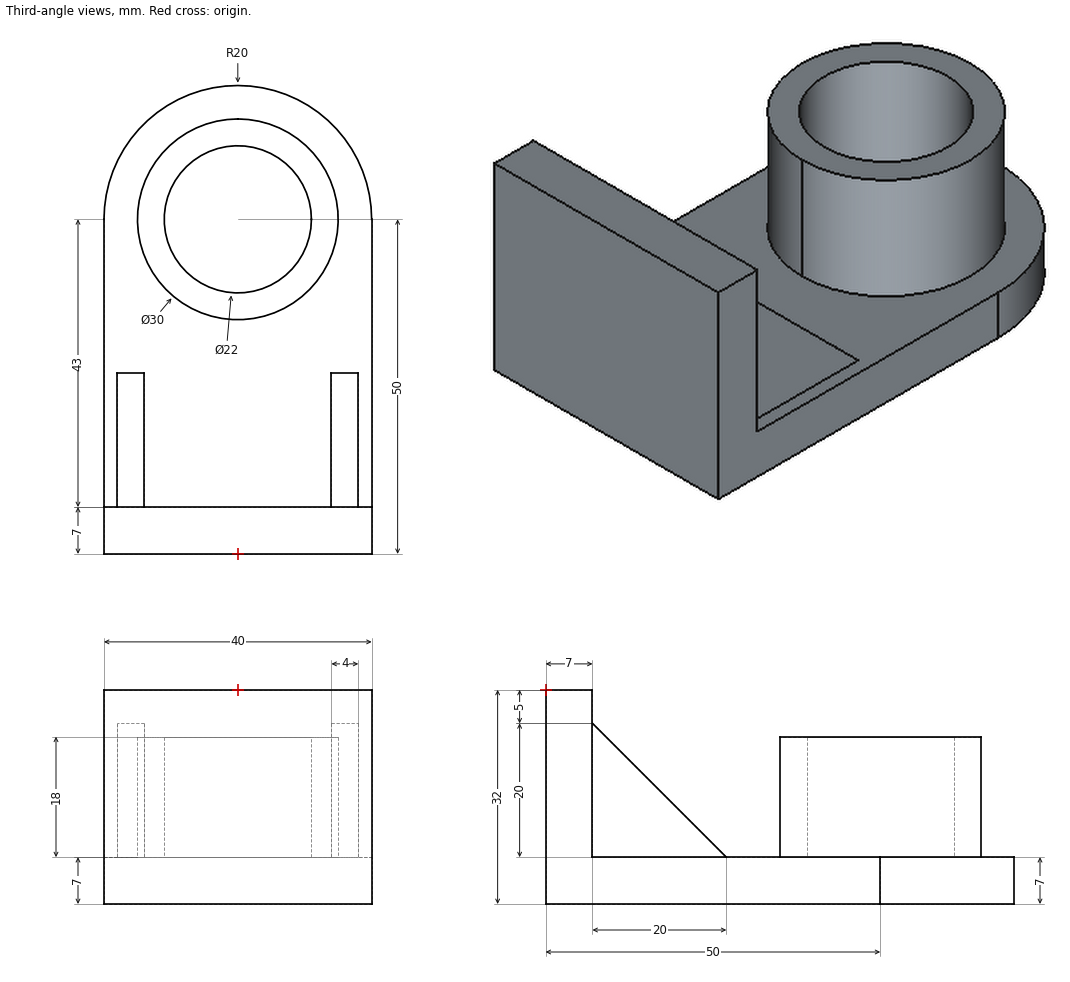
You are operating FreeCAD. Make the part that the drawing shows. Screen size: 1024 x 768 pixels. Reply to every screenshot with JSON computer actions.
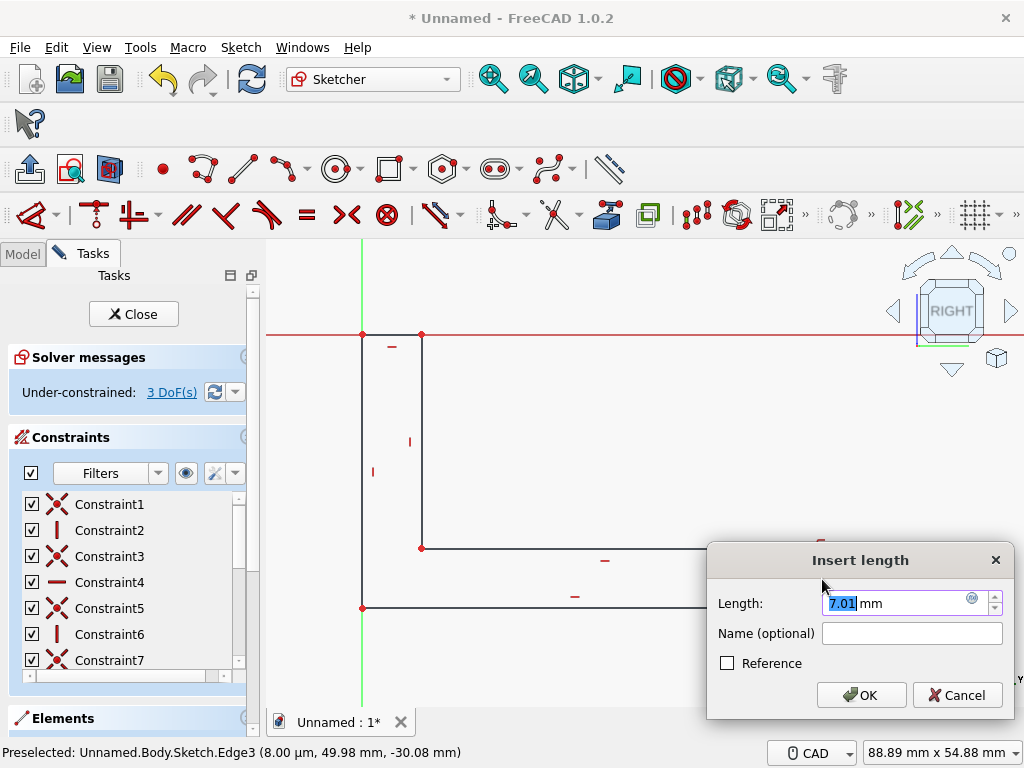
{"action": "type", "text": "7"}
{"action": "key", "text": "Return"}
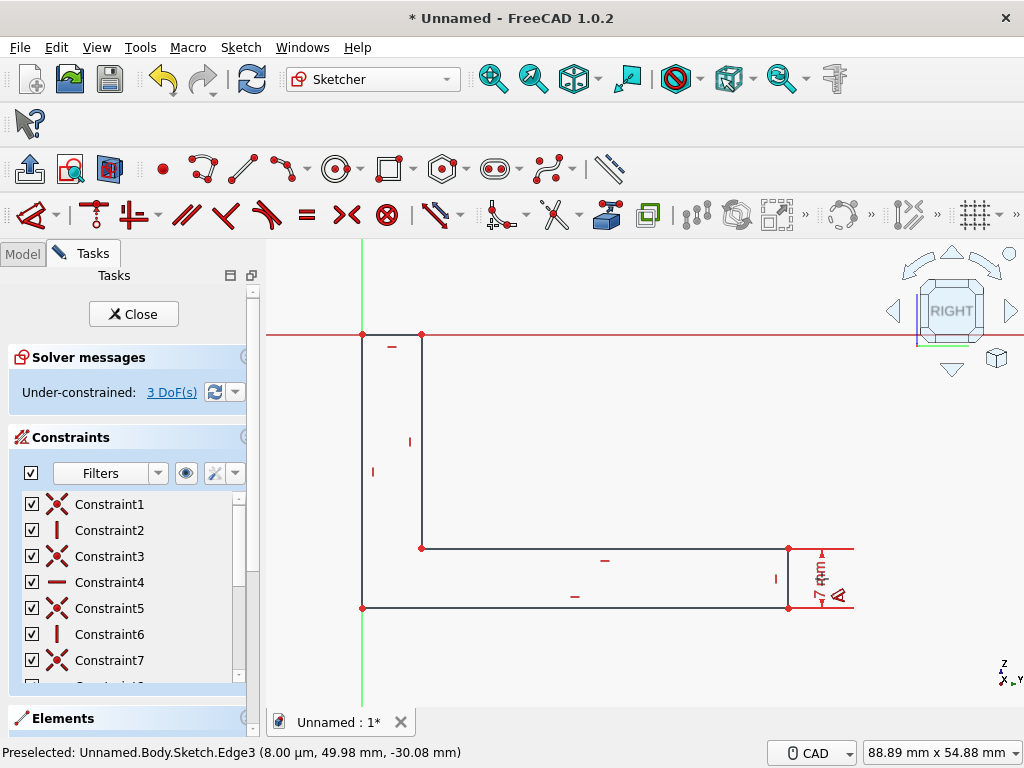
{"action": "left_click", "coordinate": [404, 335]}
{"action": "left_click", "coordinate": [392, 301]}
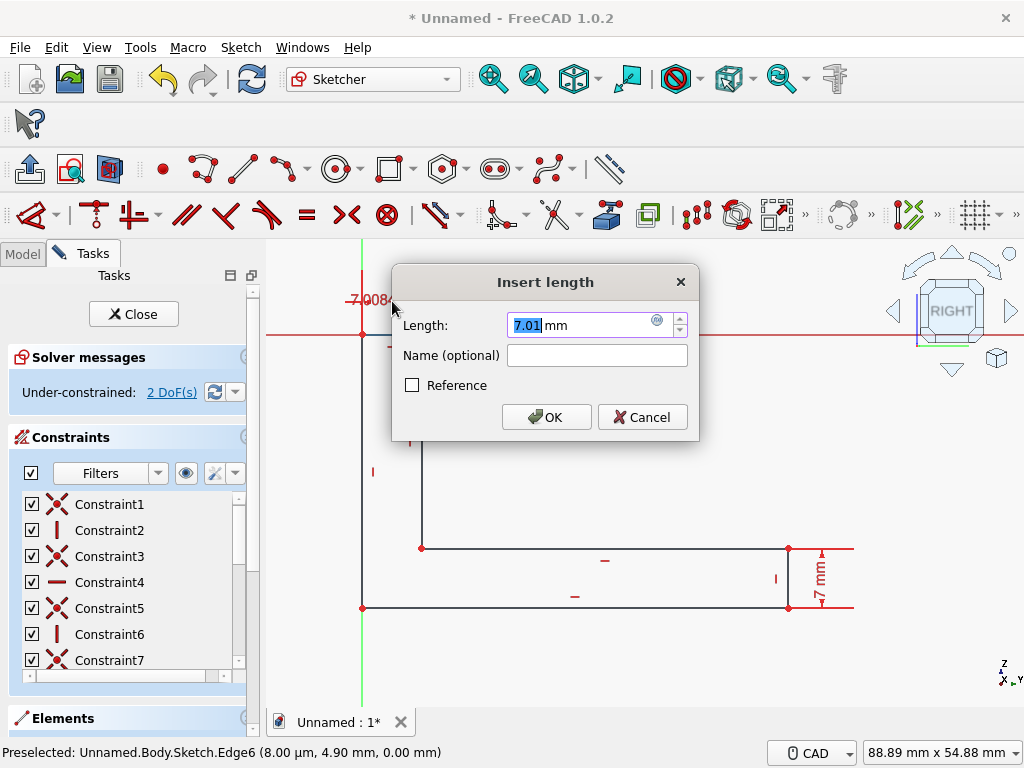
{"action": "type", "text": "7"}
{"action": "key", "text": "Return"}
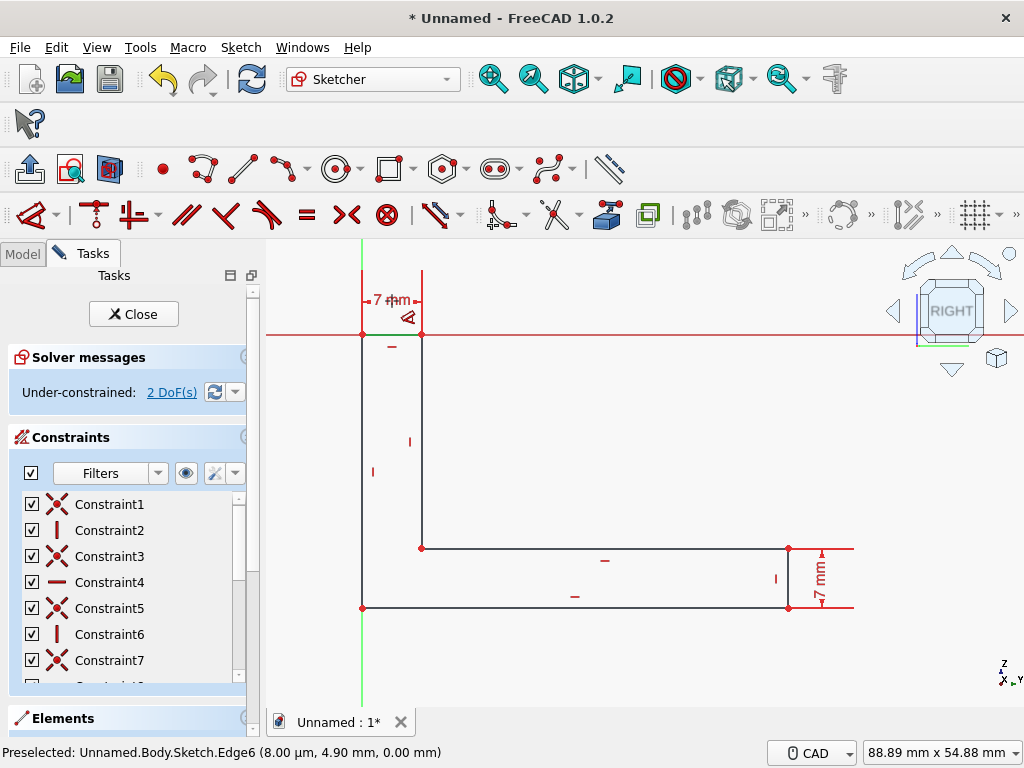
{"action": "left_click", "coordinate": [362, 417]}
{"action": "left_click", "coordinate": [328, 471]}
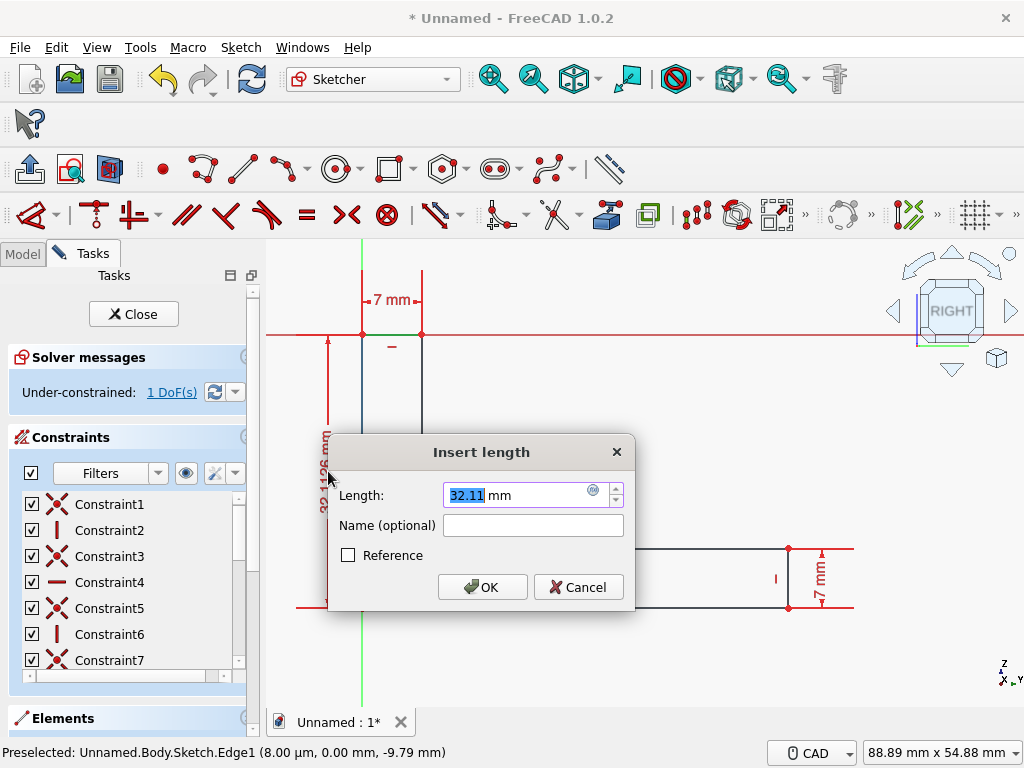
{"action": "type", "text": "32"}
{"action": "key", "text": "Return"}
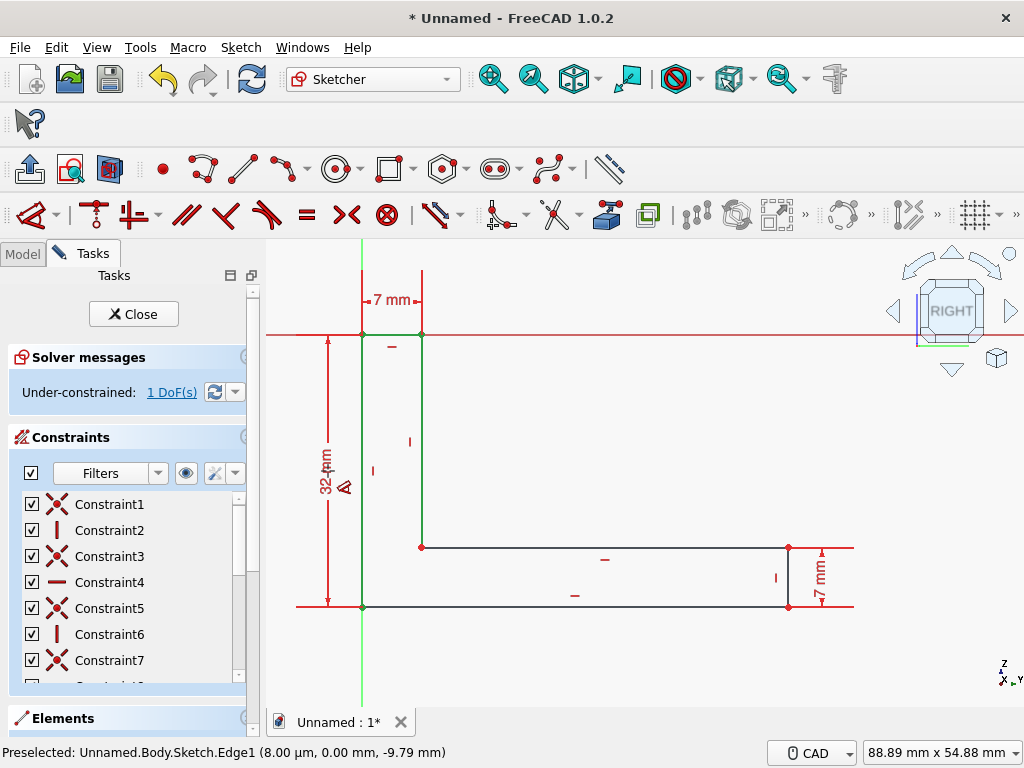
{"action": "left_click", "coordinate": [490, 607]}
{"action": "left_click", "coordinate": [575, 641]}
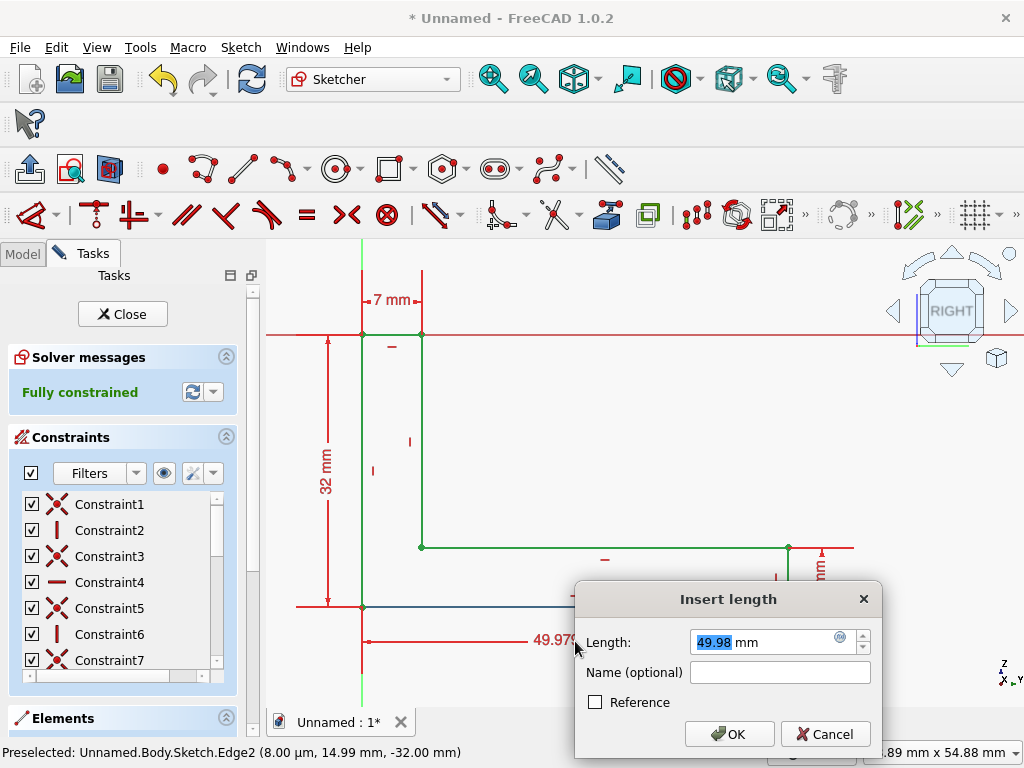
{"action": "type", "text": "50"}
{"action": "key", "text": "Return"}
{"action": "key", "text": "Escape"}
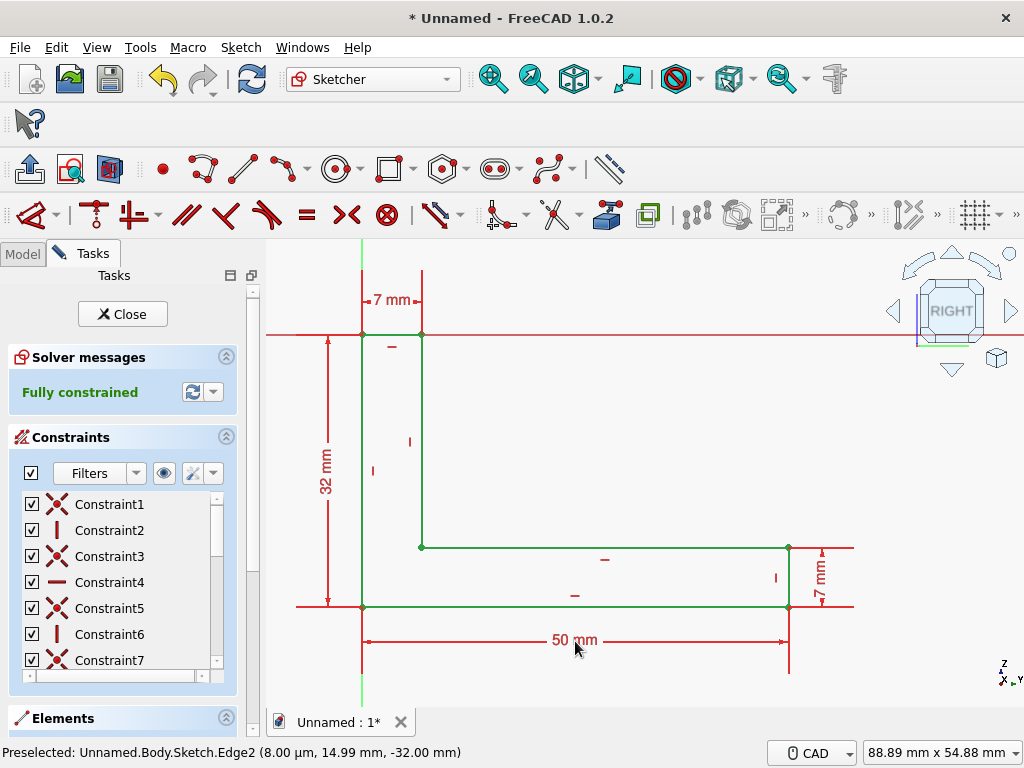
{"action": "left_click", "coordinate": [123, 314]}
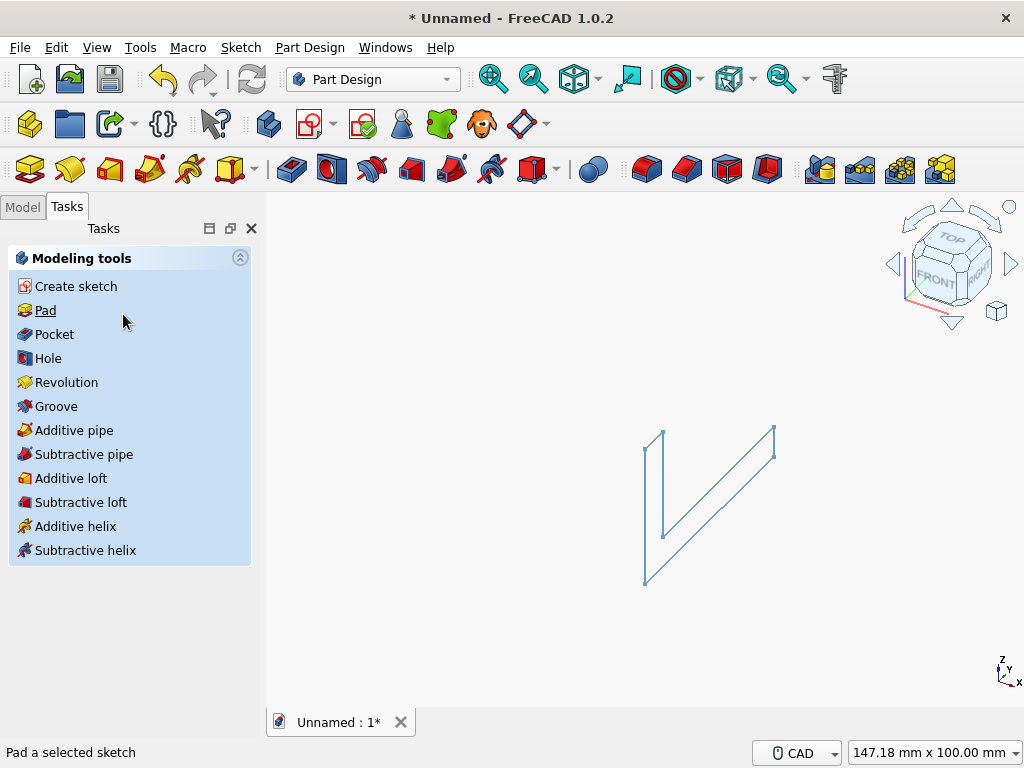
{"action": "left_click", "coordinate": [30, 170]}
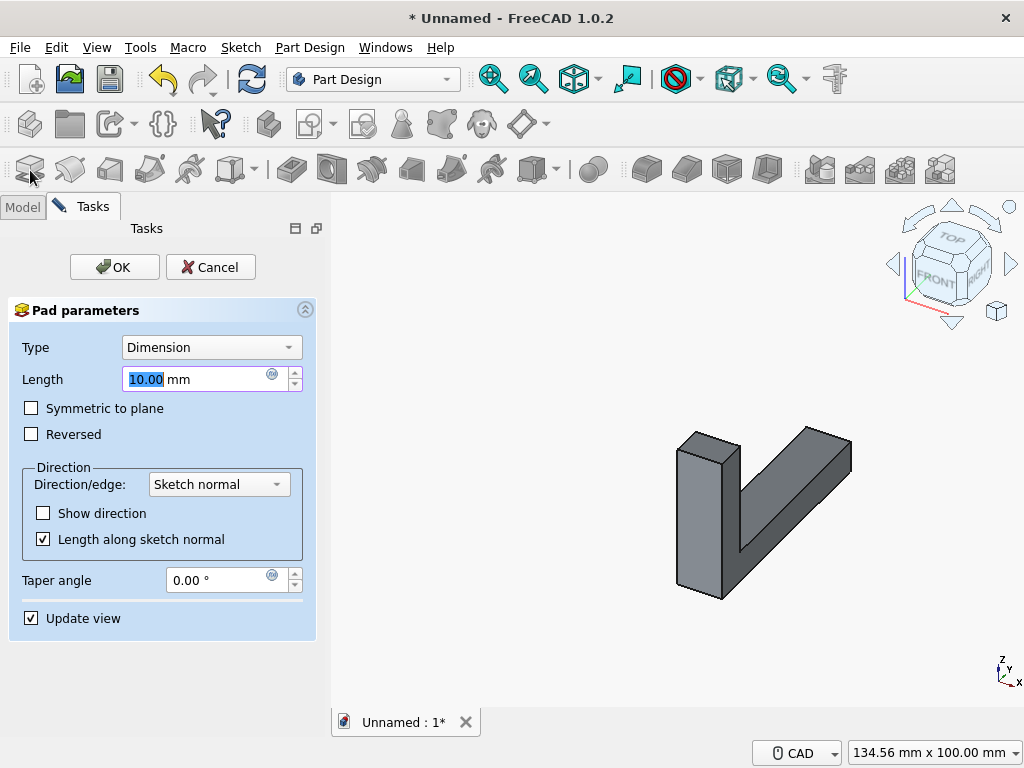
{"action": "type", "text": "40"}
{"action": "key", "text": "Tab"}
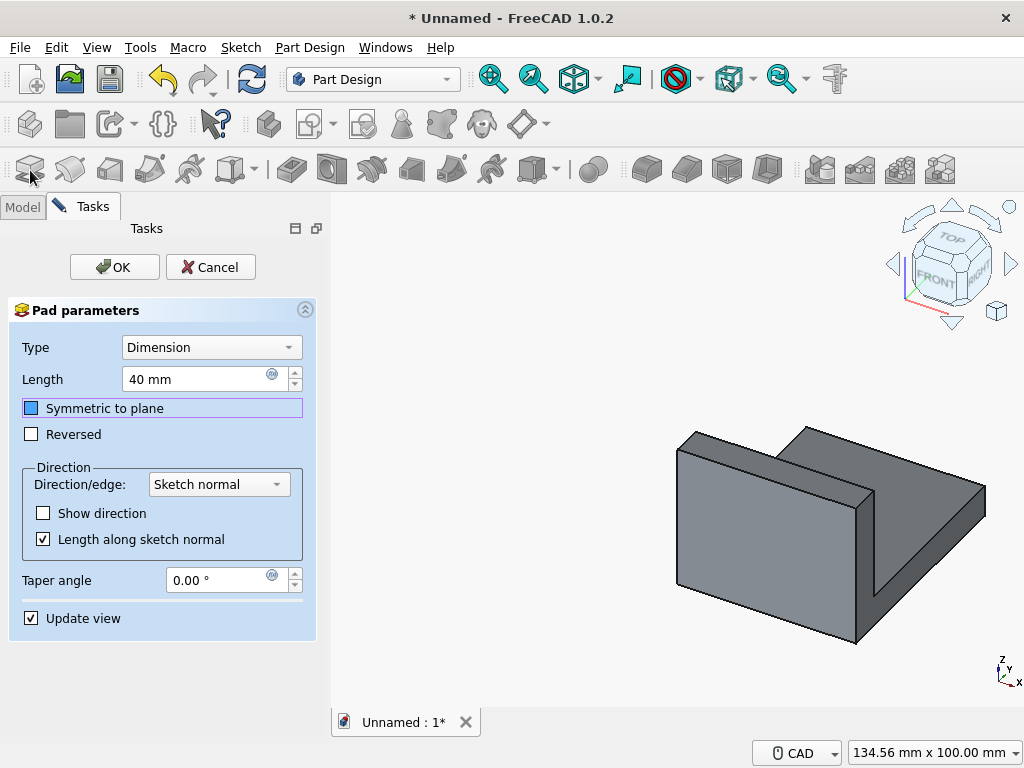
{"action": "left_click", "coordinate": [30, 408]}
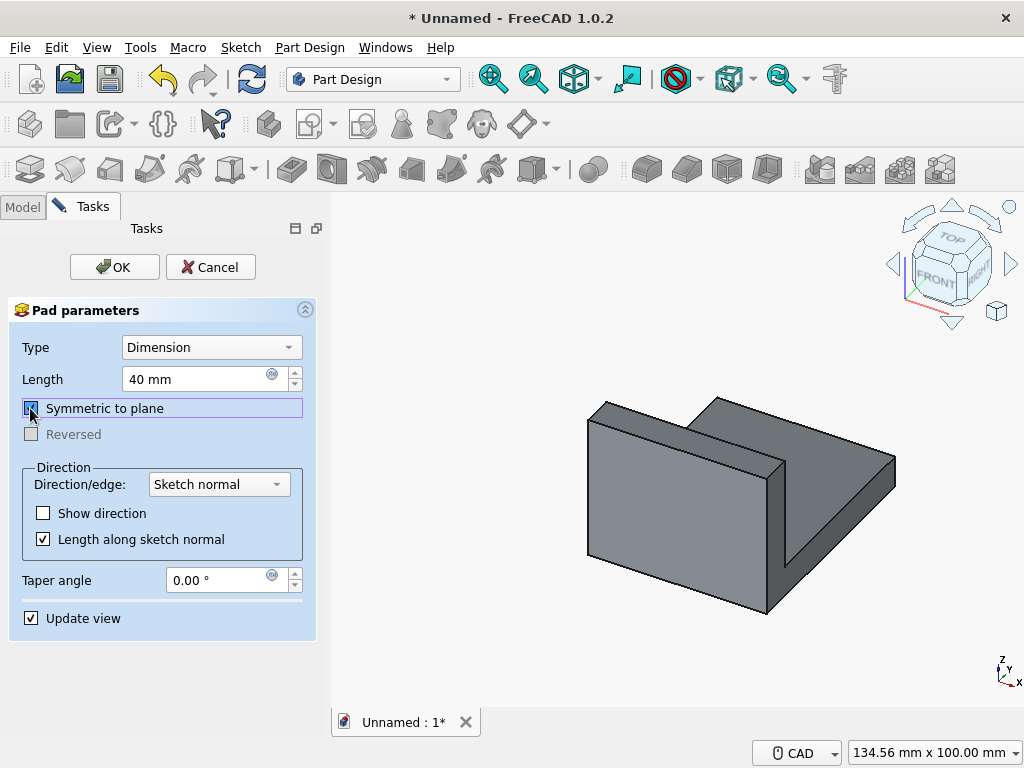
{"action": "left_click", "coordinate": [115, 267]}